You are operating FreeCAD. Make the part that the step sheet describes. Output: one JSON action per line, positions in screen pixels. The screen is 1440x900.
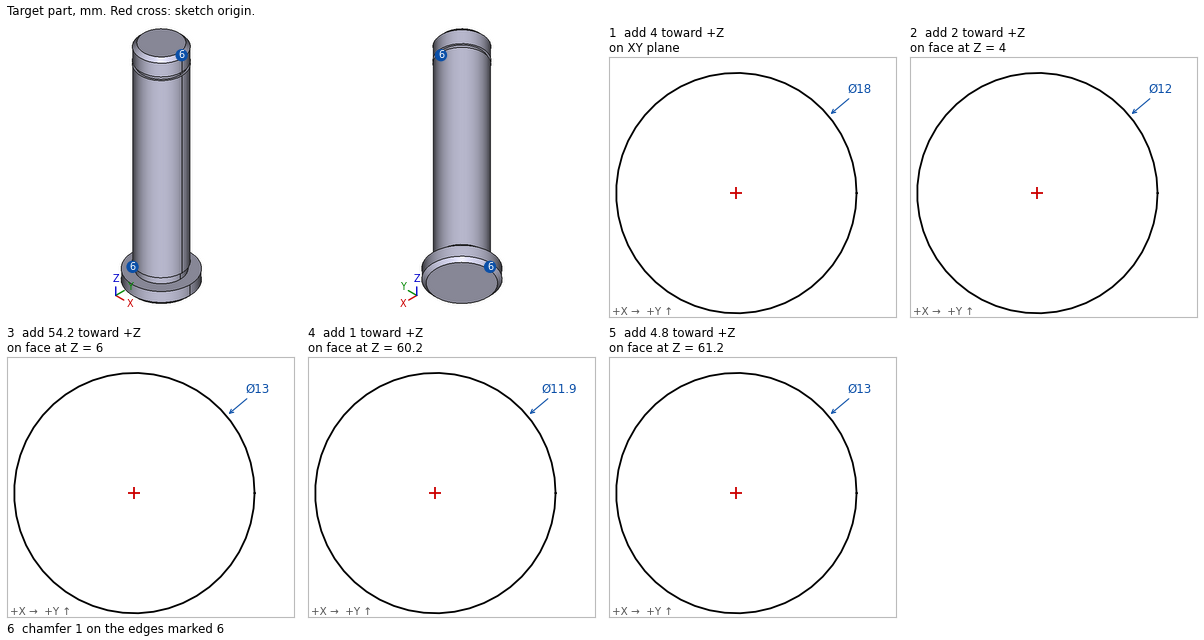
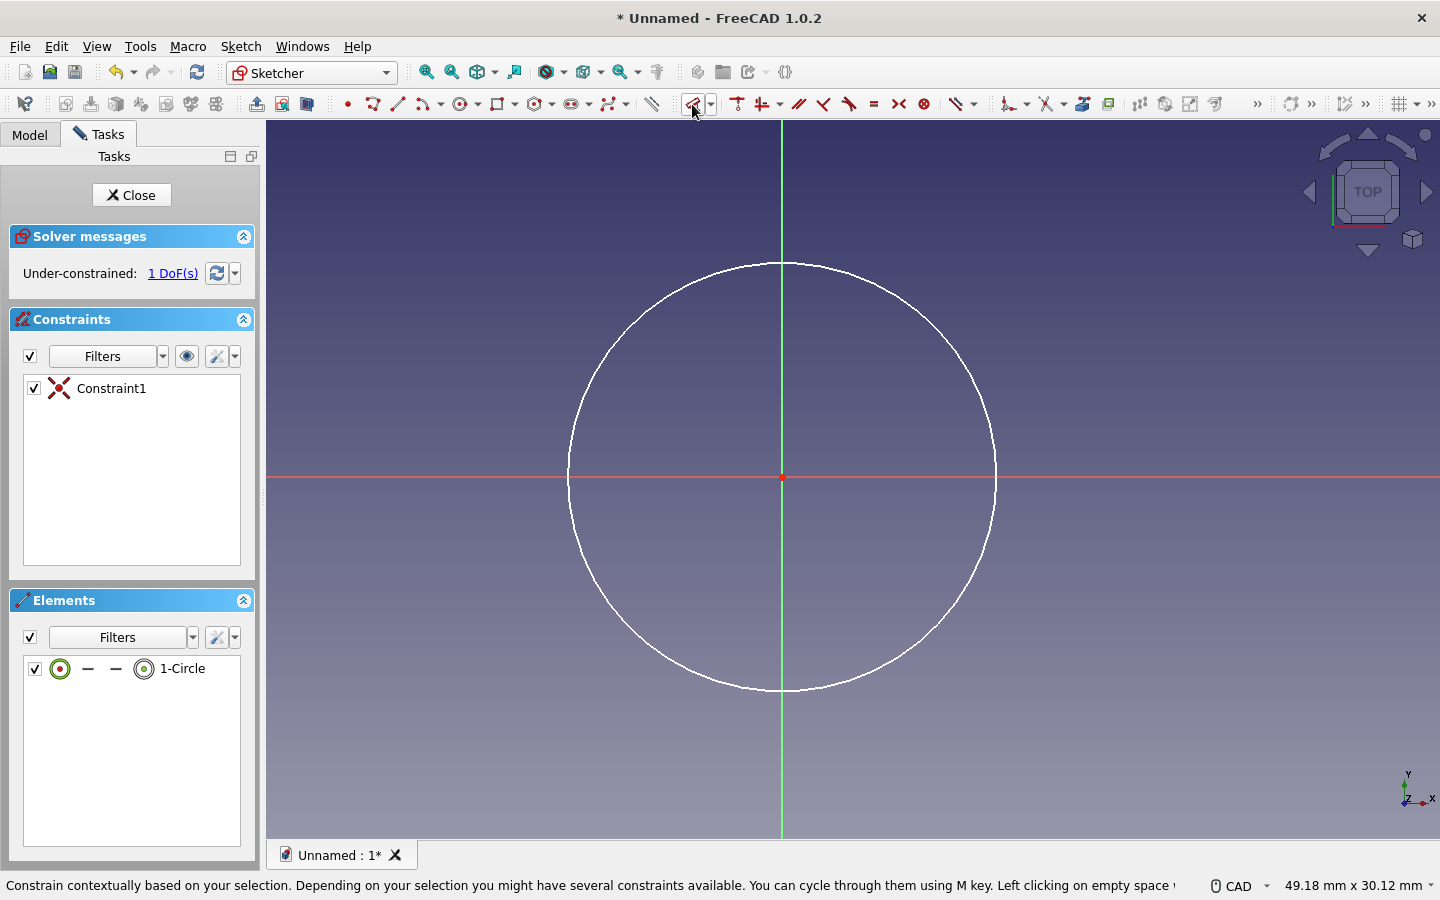
{"action": "left_click", "coordinate": [933, 325]}
{"action": "left_click", "coordinate": [956, 302]}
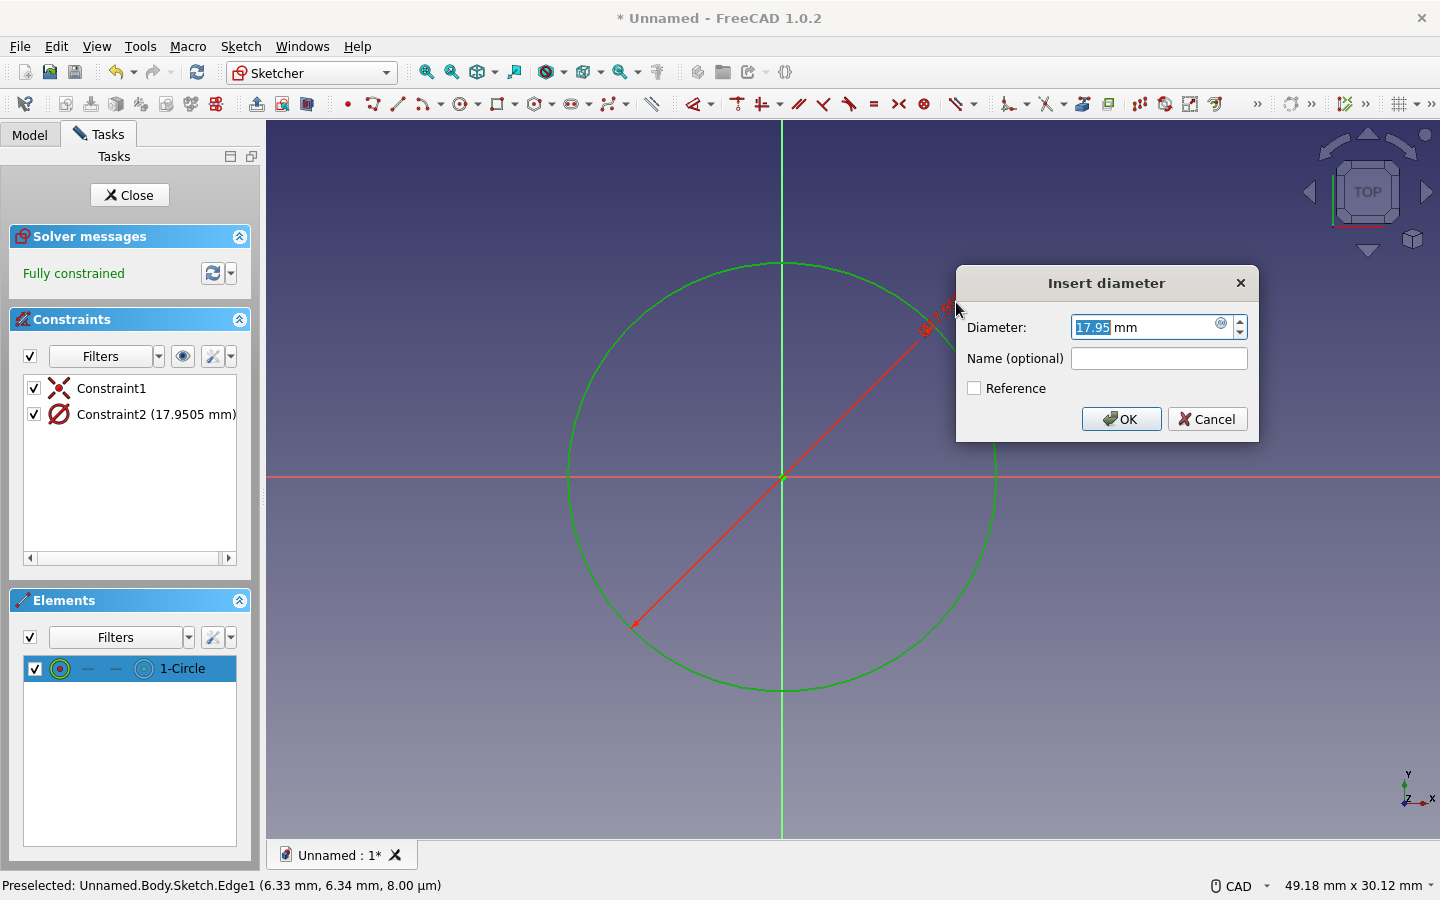
{"action": "type", "text": "18"}
{"action": "key", "text": "Return"}
{"action": "key", "text": "Escape"}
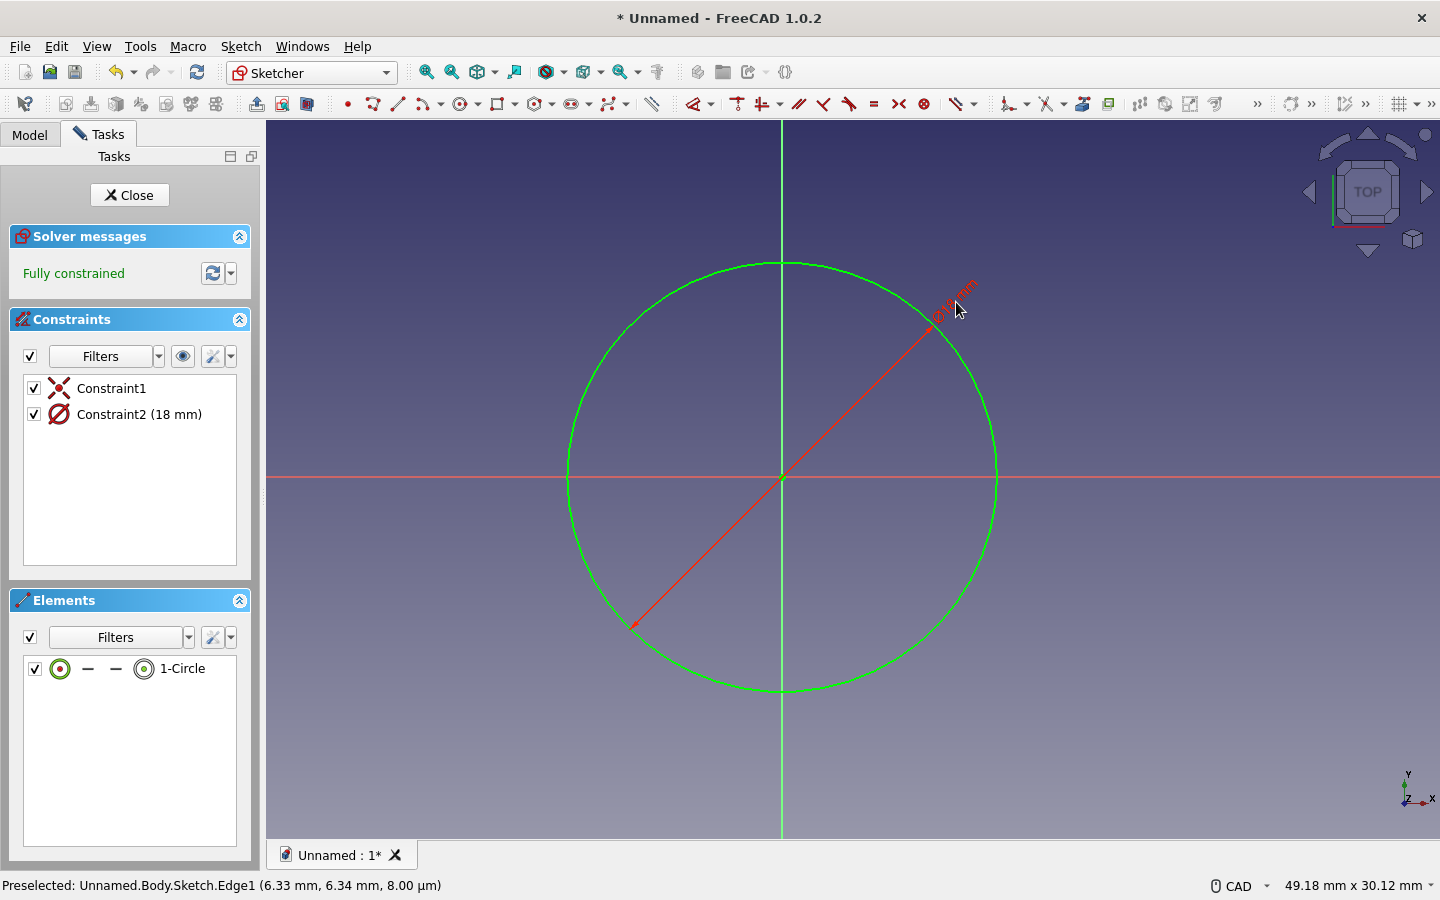
{"action": "left_click", "coordinate": [130, 195]}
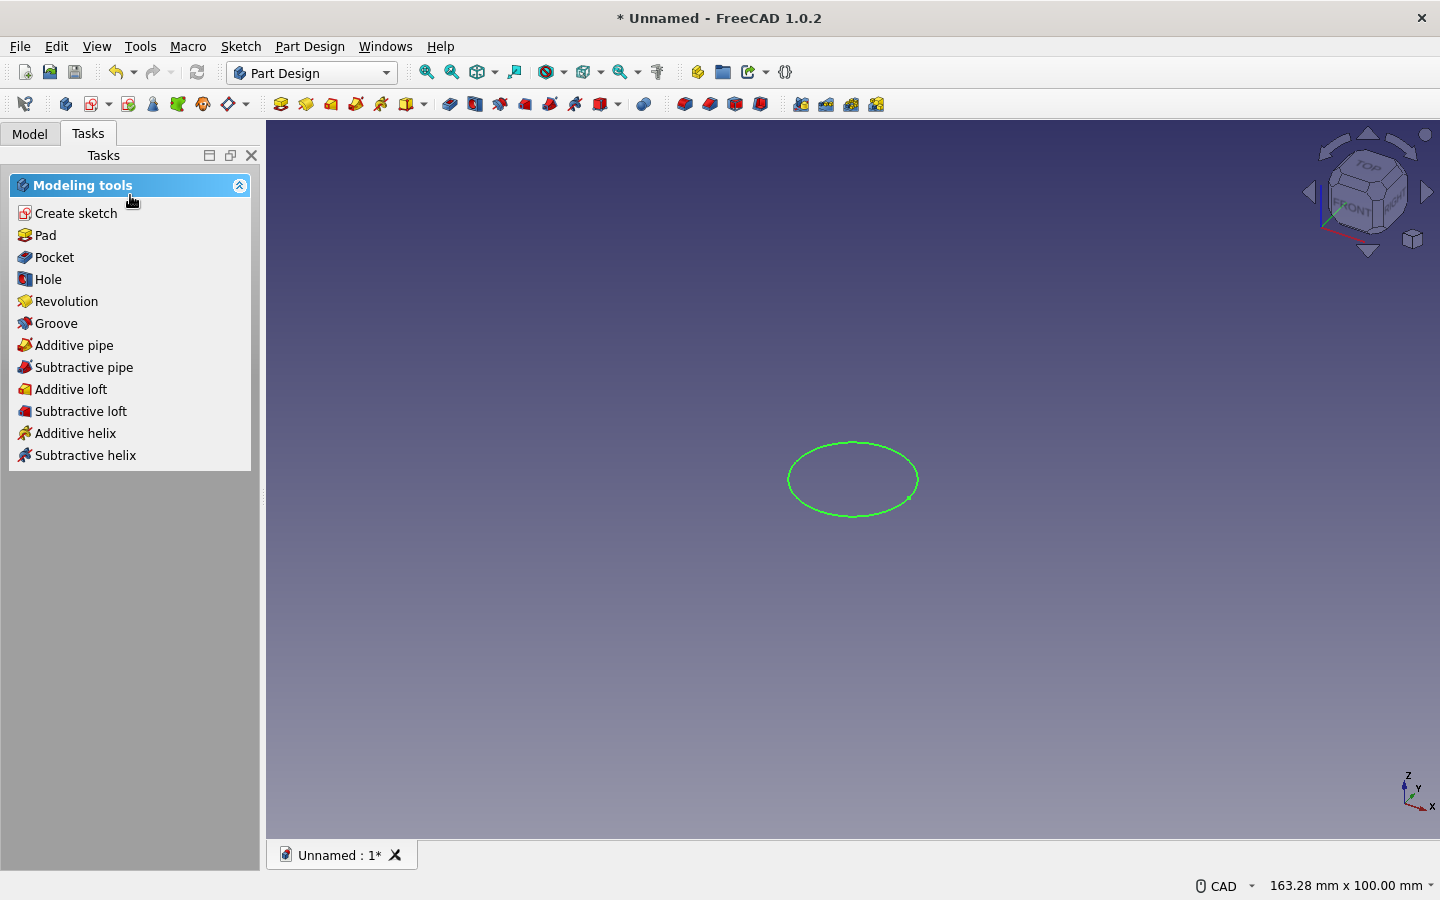
{"action": "left_click", "coordinate": [281, 104]}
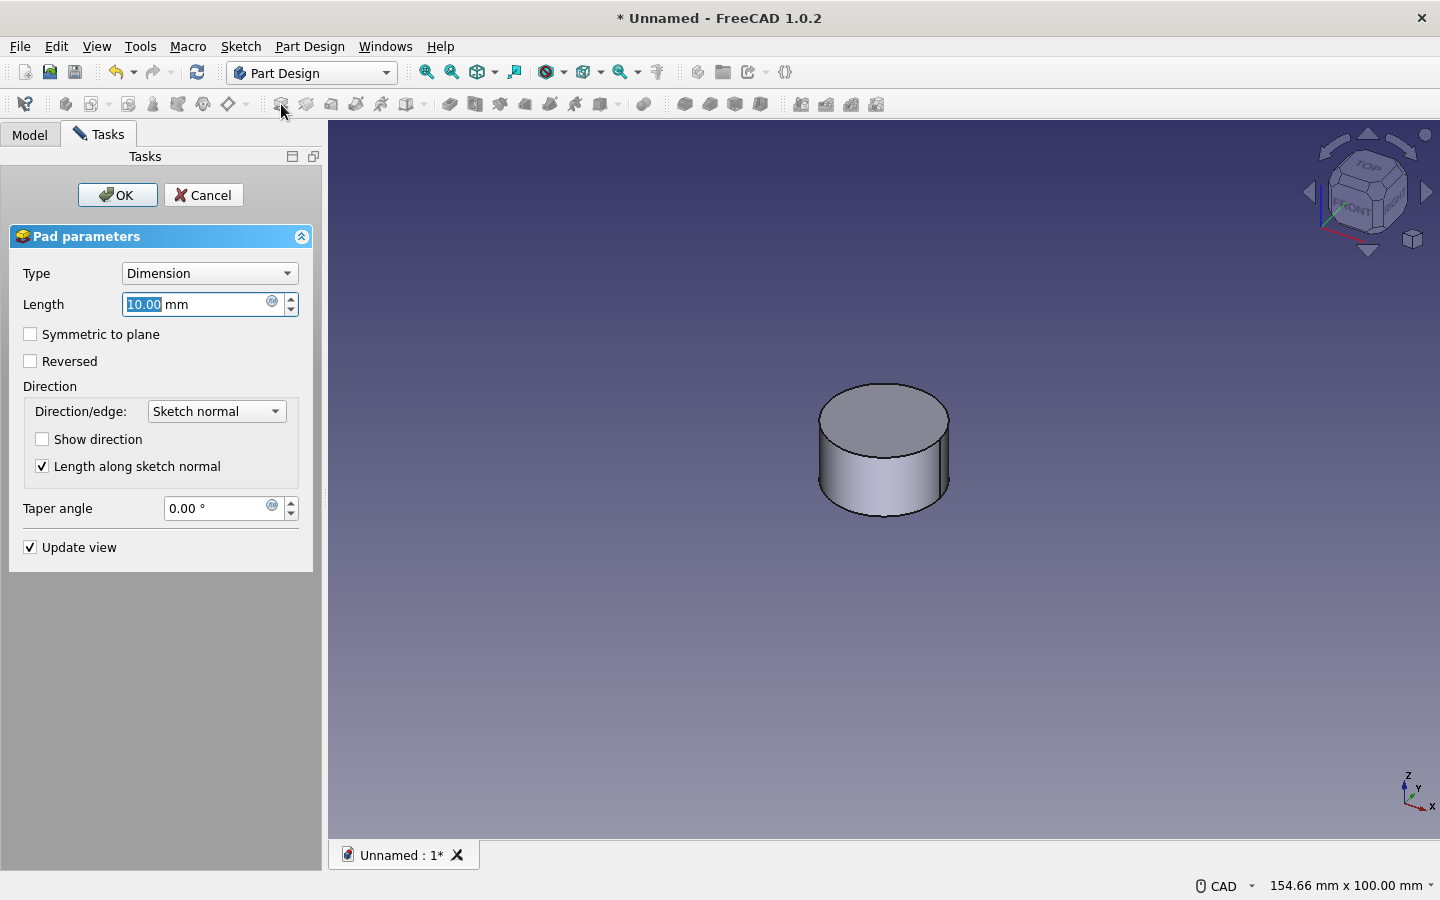
{"action": "type", "text": "4"}
{"action": "key", "text": "Tab"}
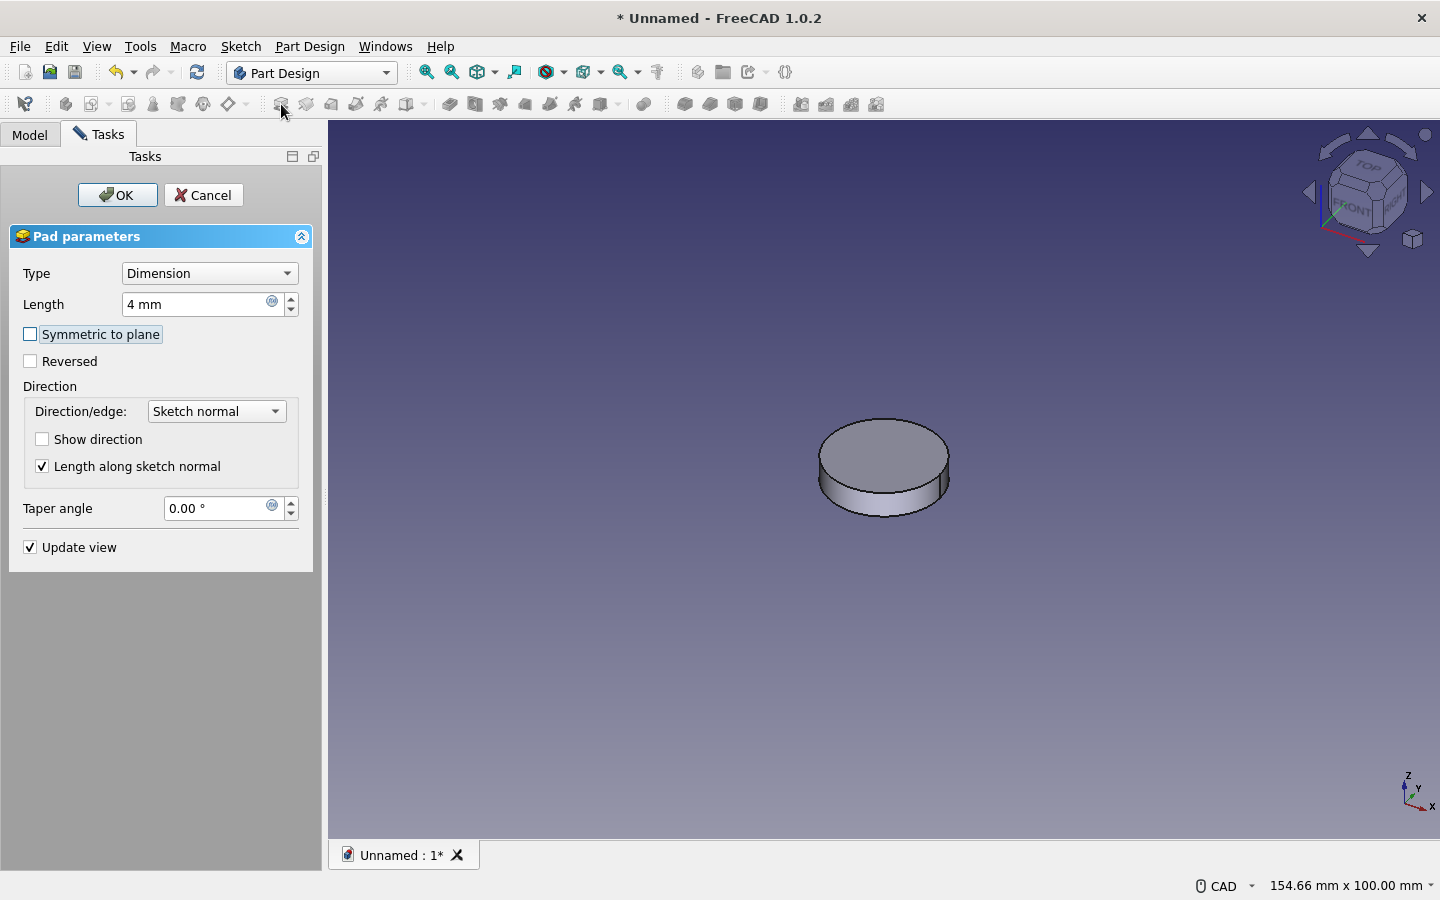
{"action": "left_click", "coordinate": [118, 195]}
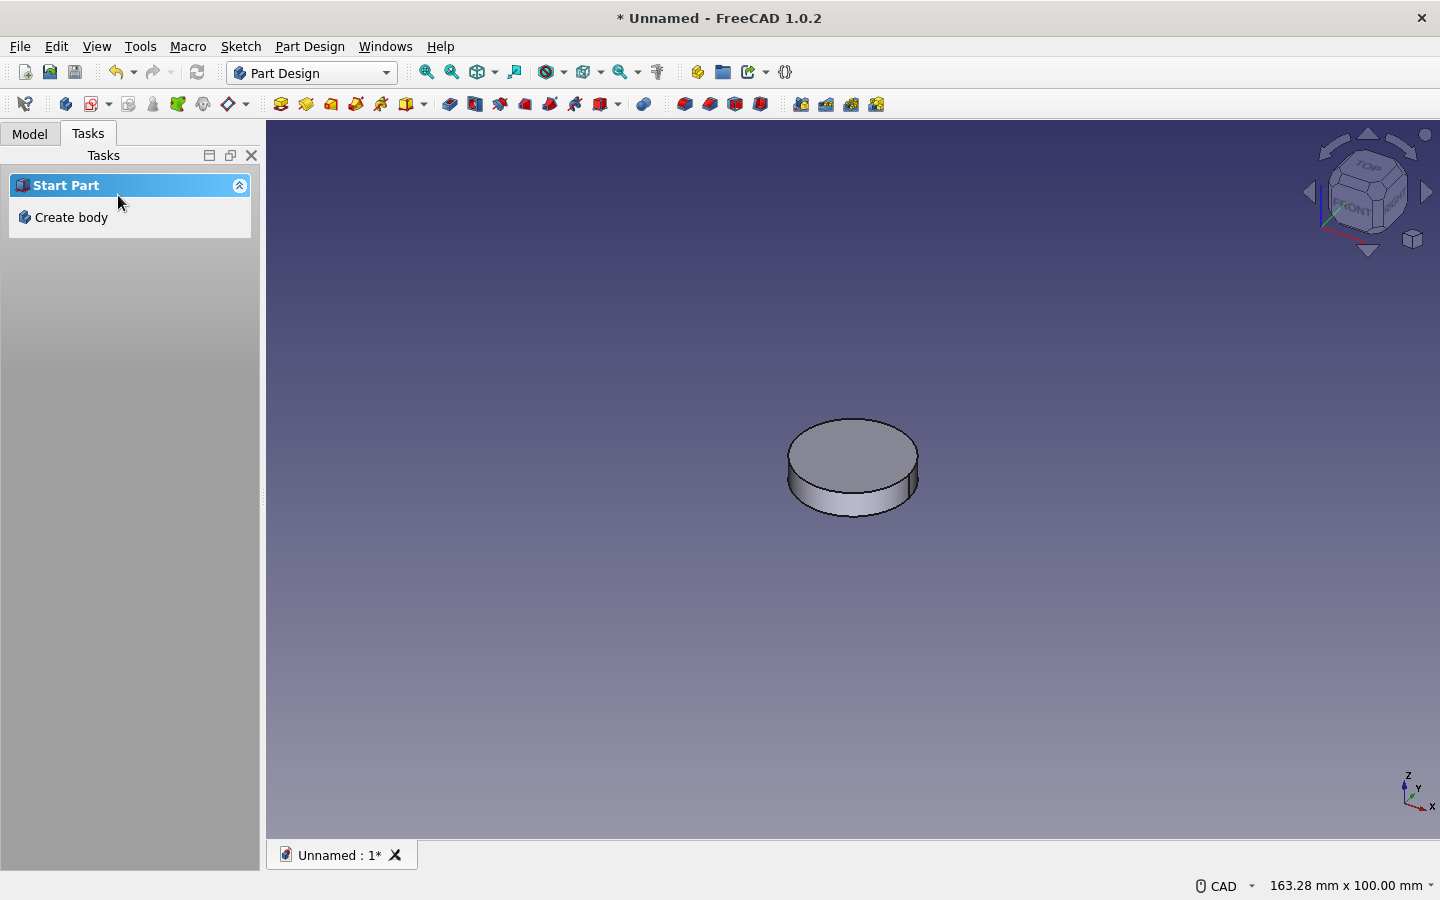
{"action": "left_click", "coordinate": [427, 72]}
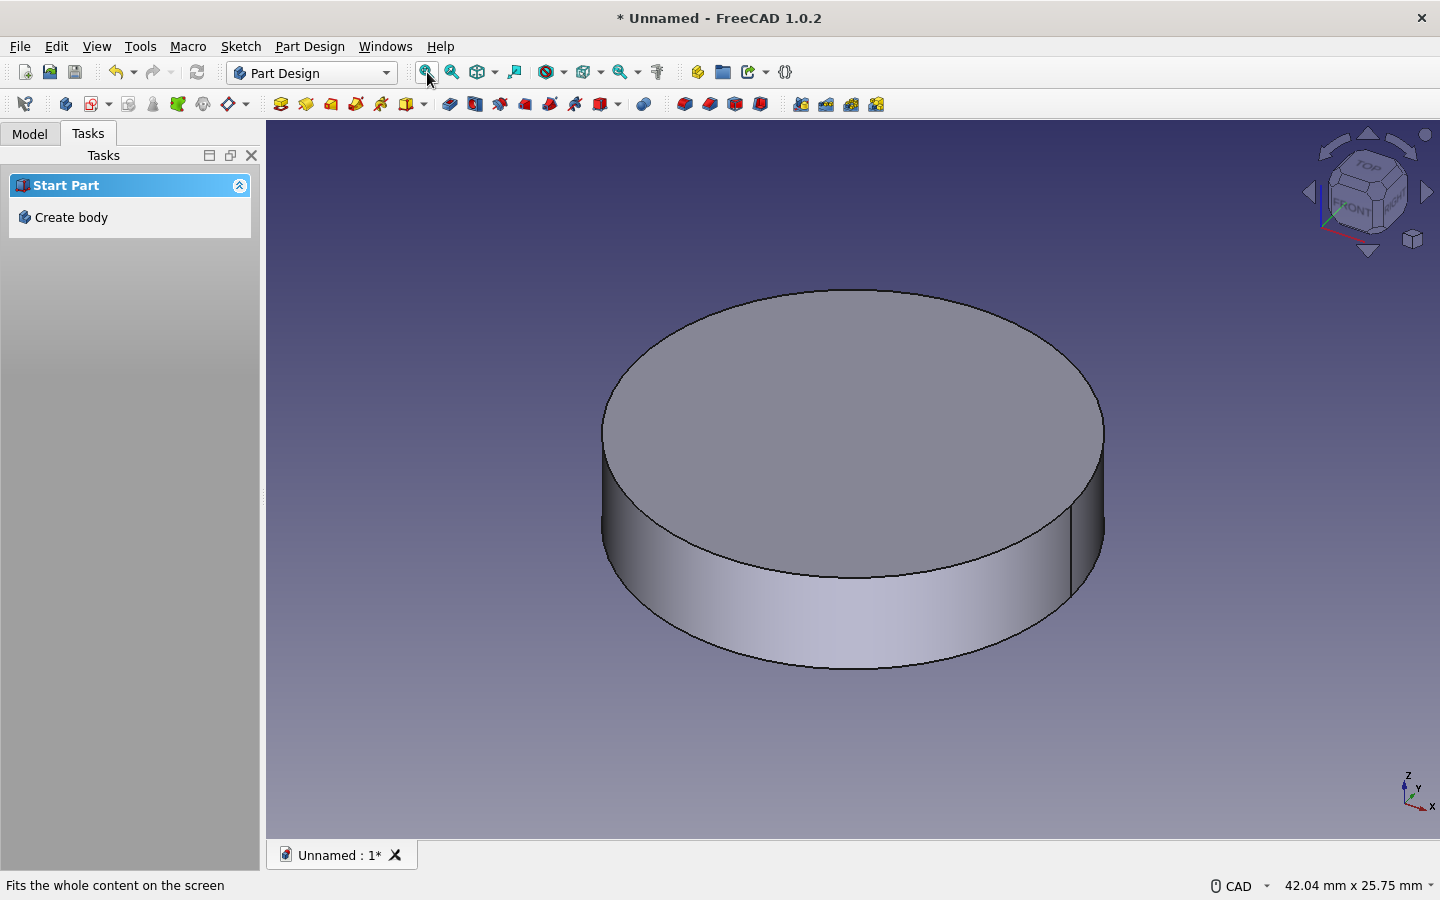
{"action": "left_click", "coordinate": [853, 433]}